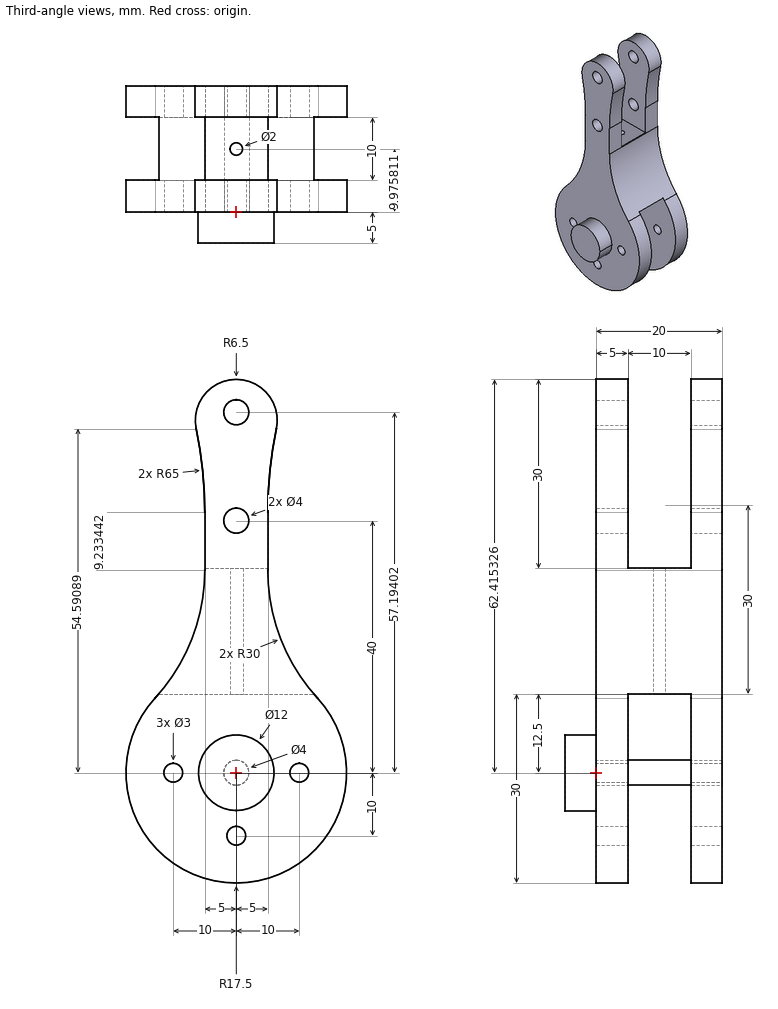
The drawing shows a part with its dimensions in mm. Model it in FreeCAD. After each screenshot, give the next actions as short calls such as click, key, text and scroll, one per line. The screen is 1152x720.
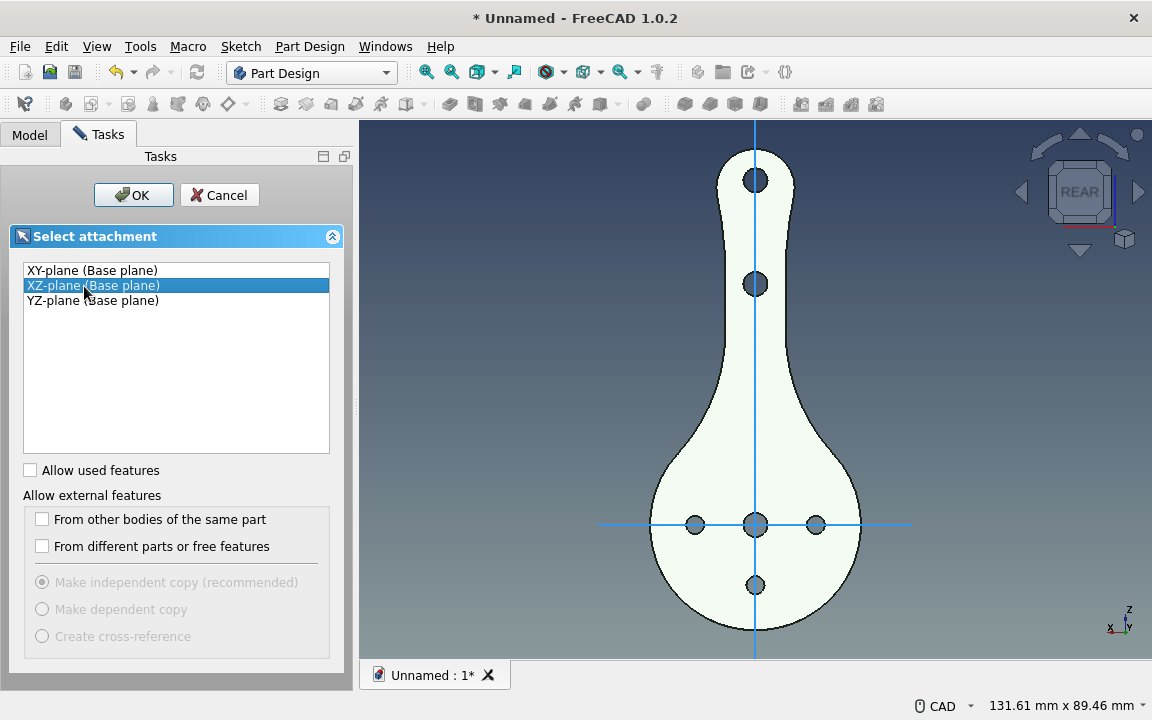
click(134, 195)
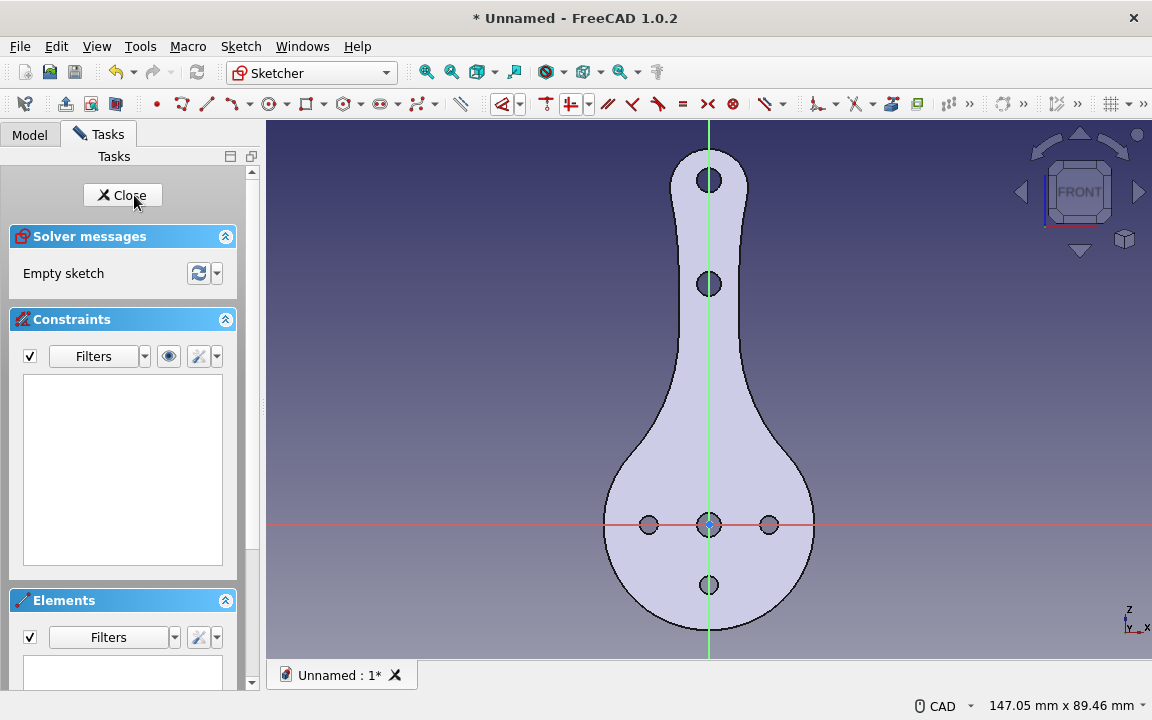
scroll(726, 559, up, 8)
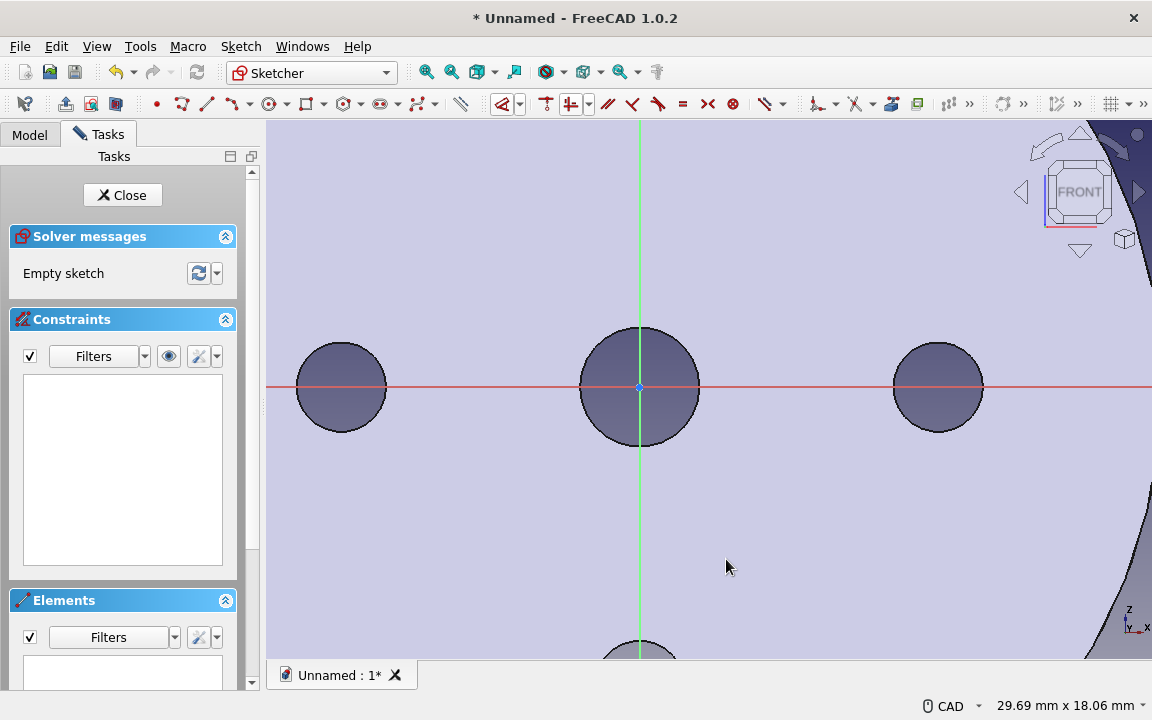
key(g)
key(c)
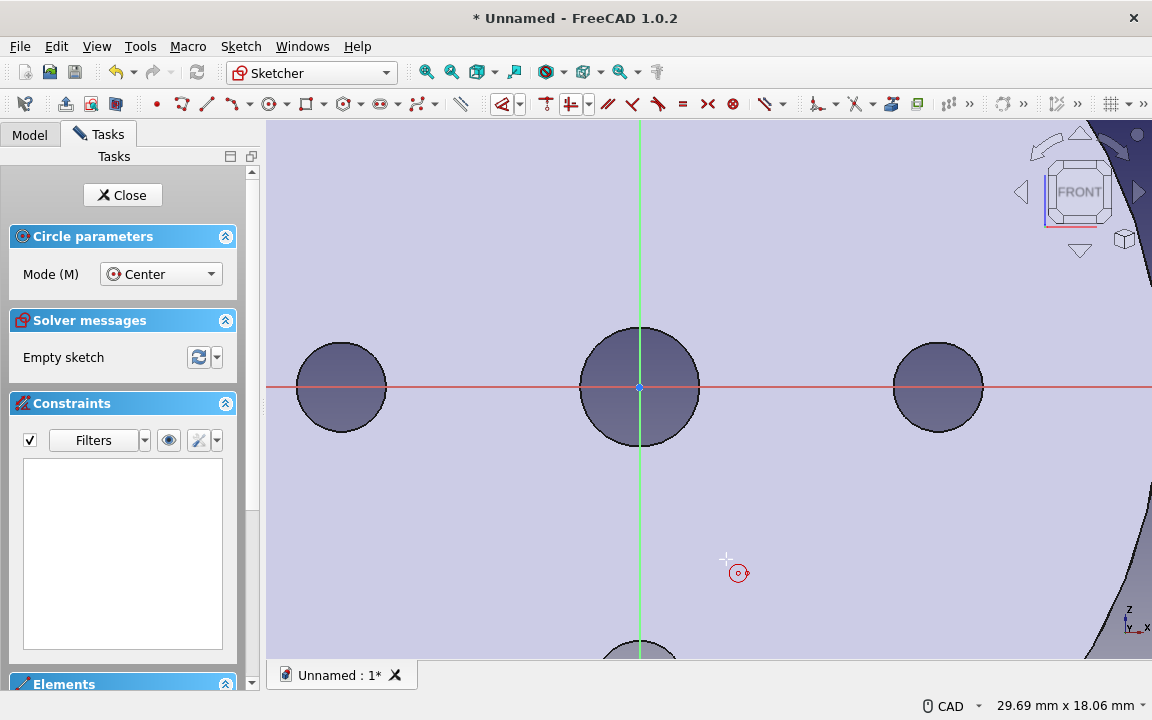
click(640, 387)
click(766, 260)
key(Escape)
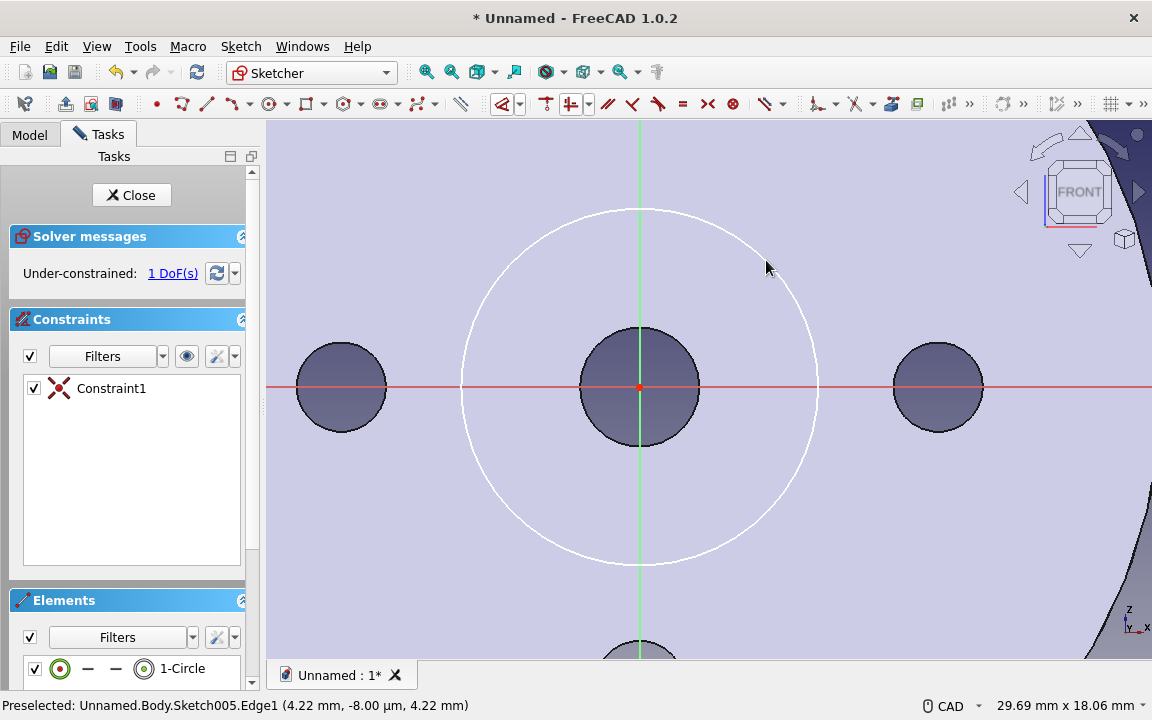
click(766, 261)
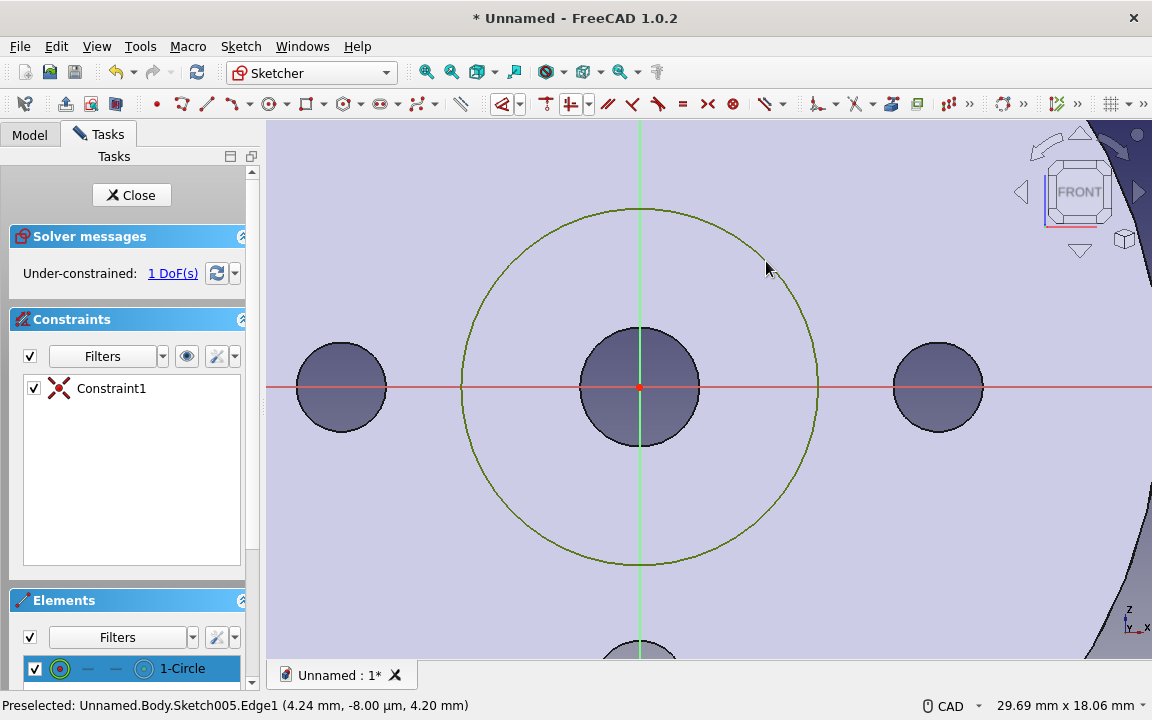
click(520, 104)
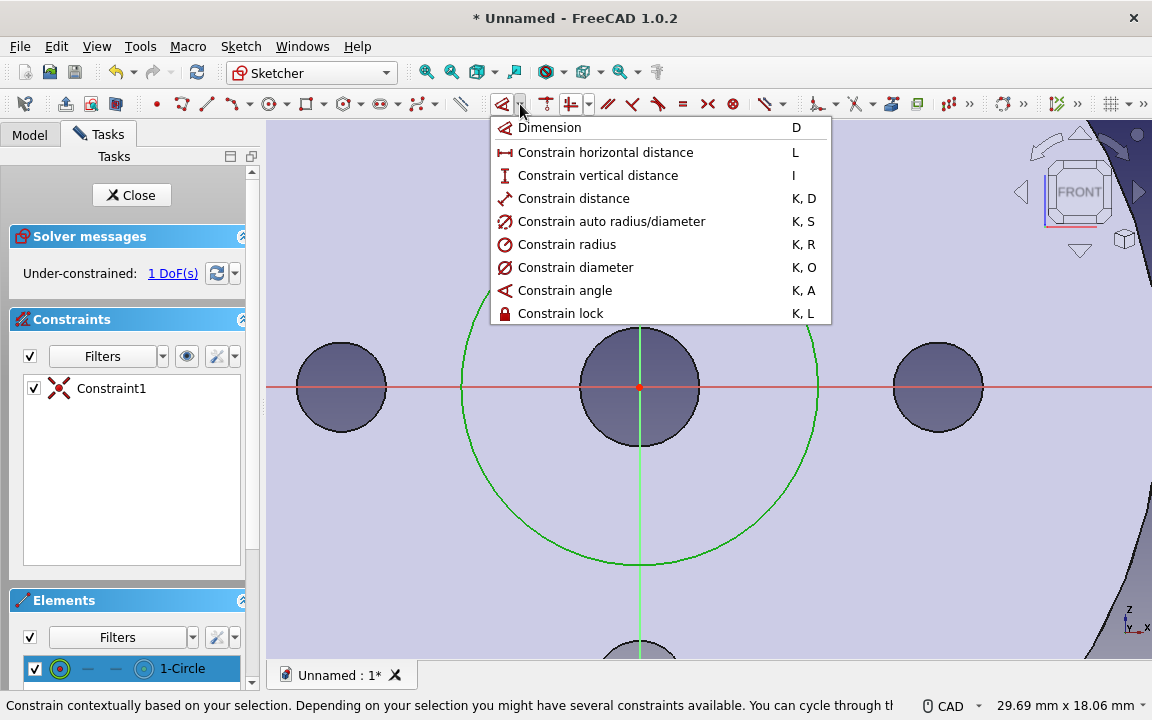
click(661, 268)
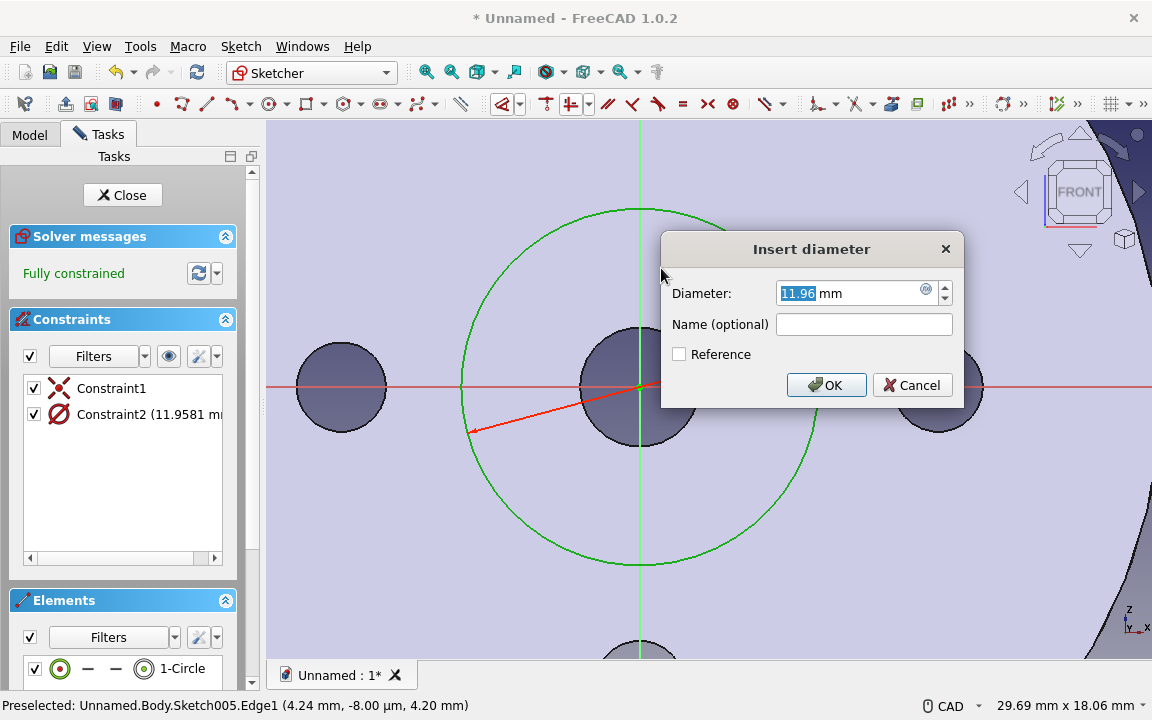
text(12)
key(Return)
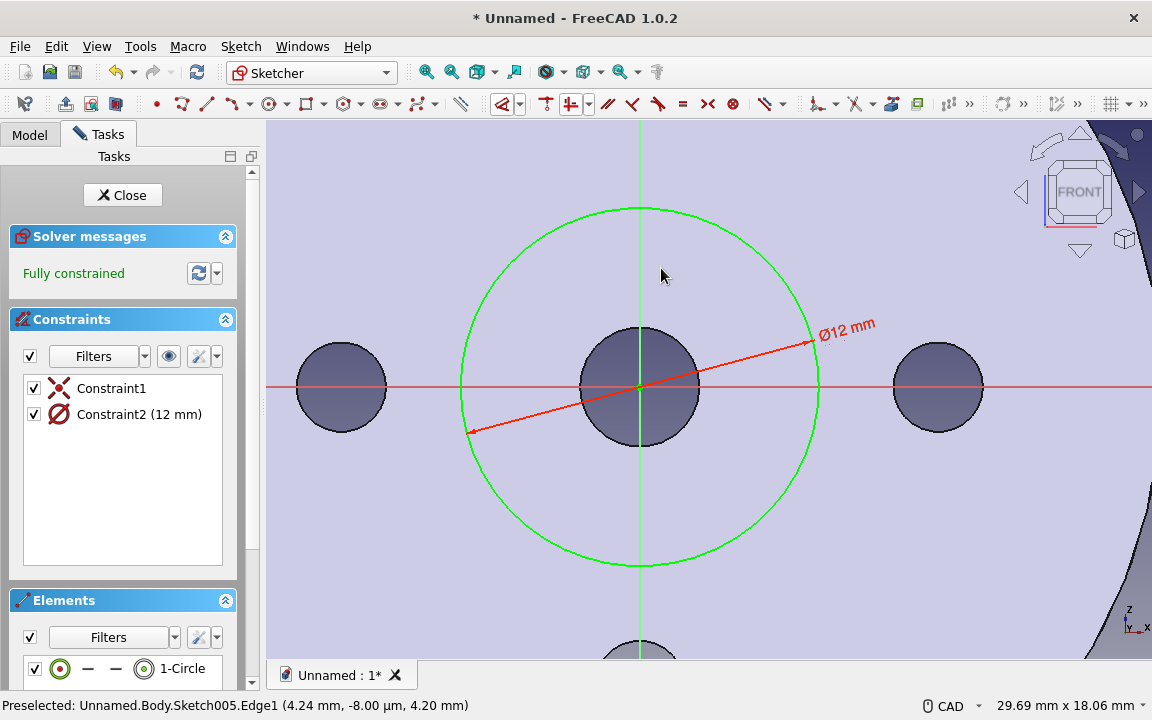
click(123, 195)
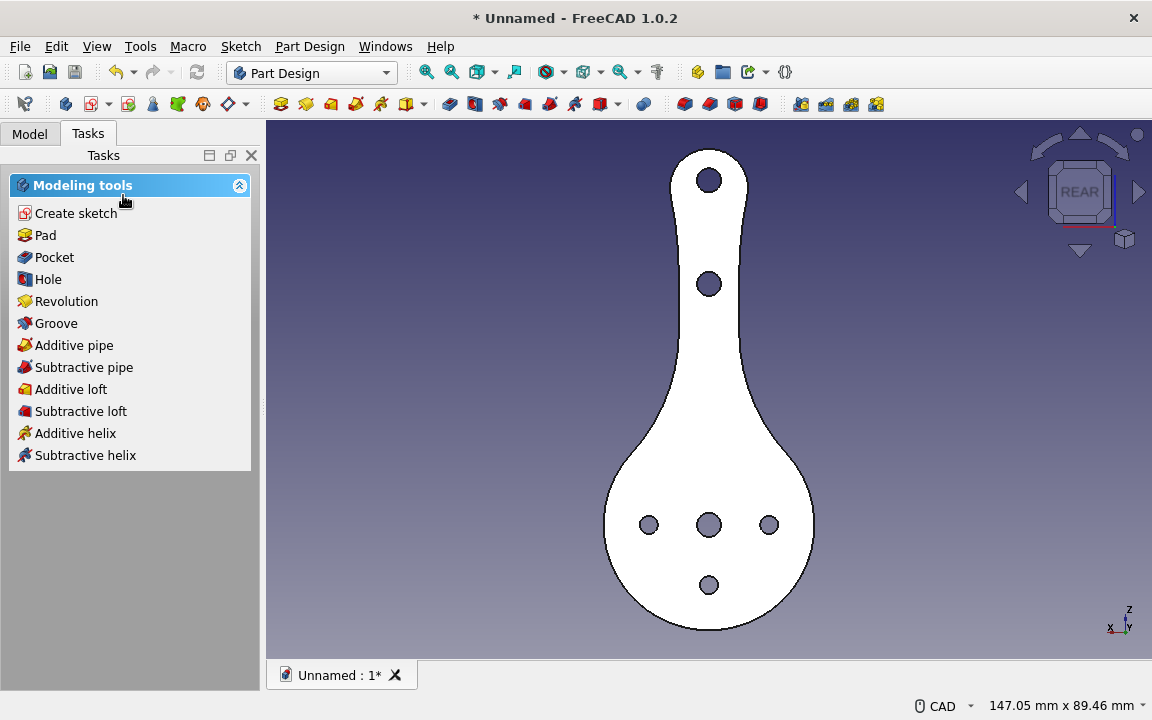
click(281, 104)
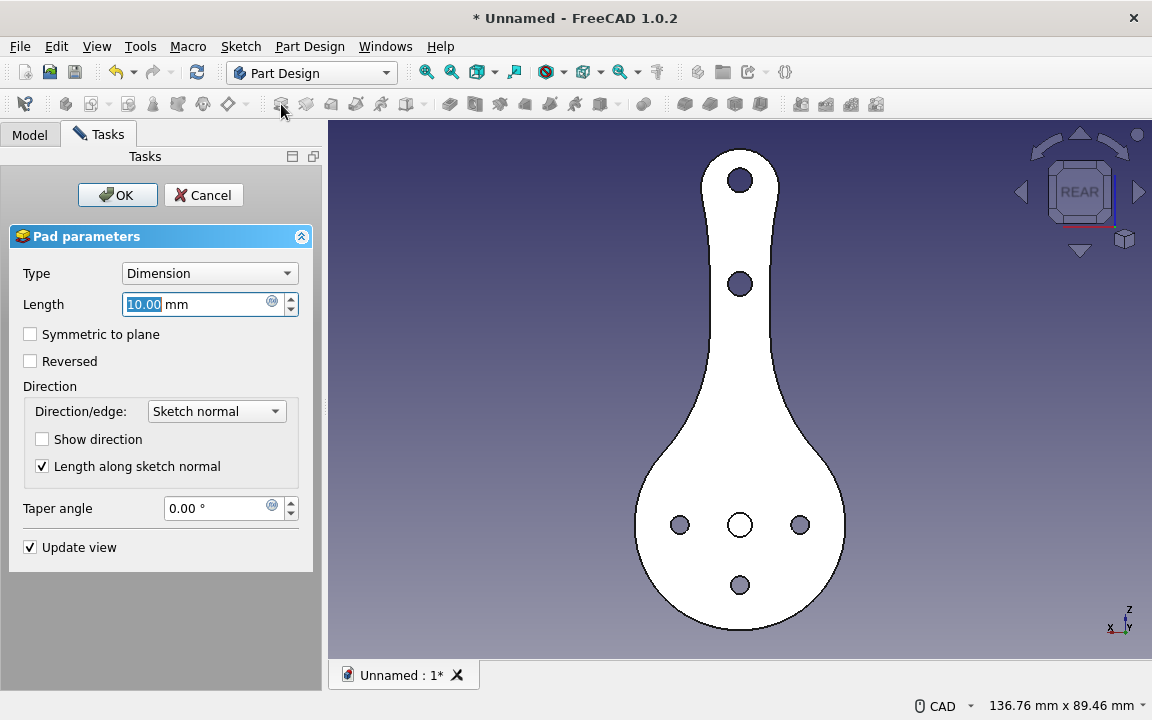
text(5)
key(Tab)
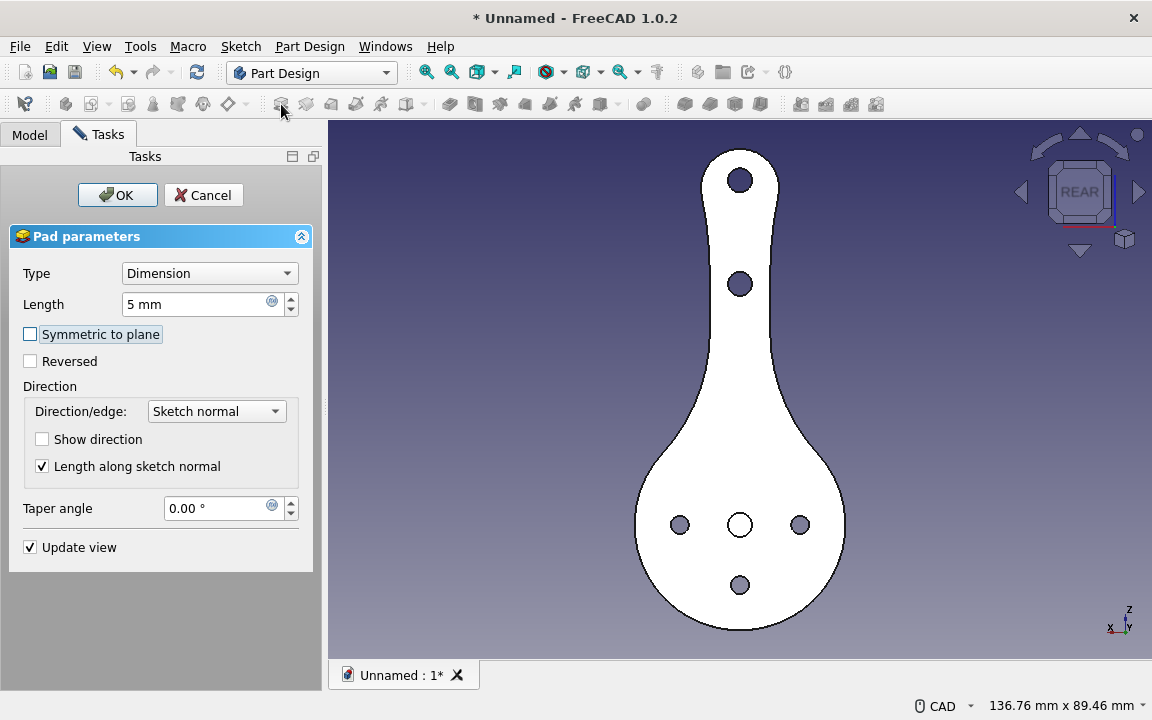
click(118, 195)